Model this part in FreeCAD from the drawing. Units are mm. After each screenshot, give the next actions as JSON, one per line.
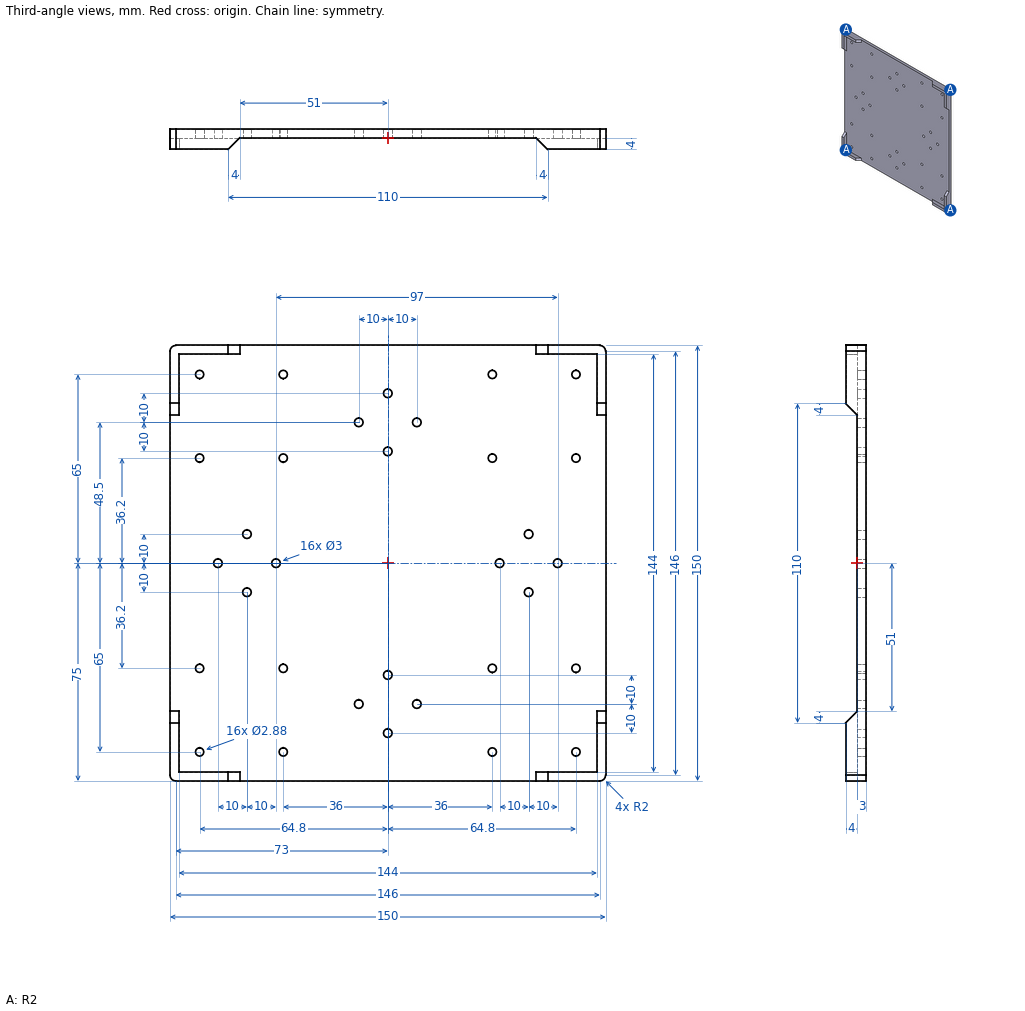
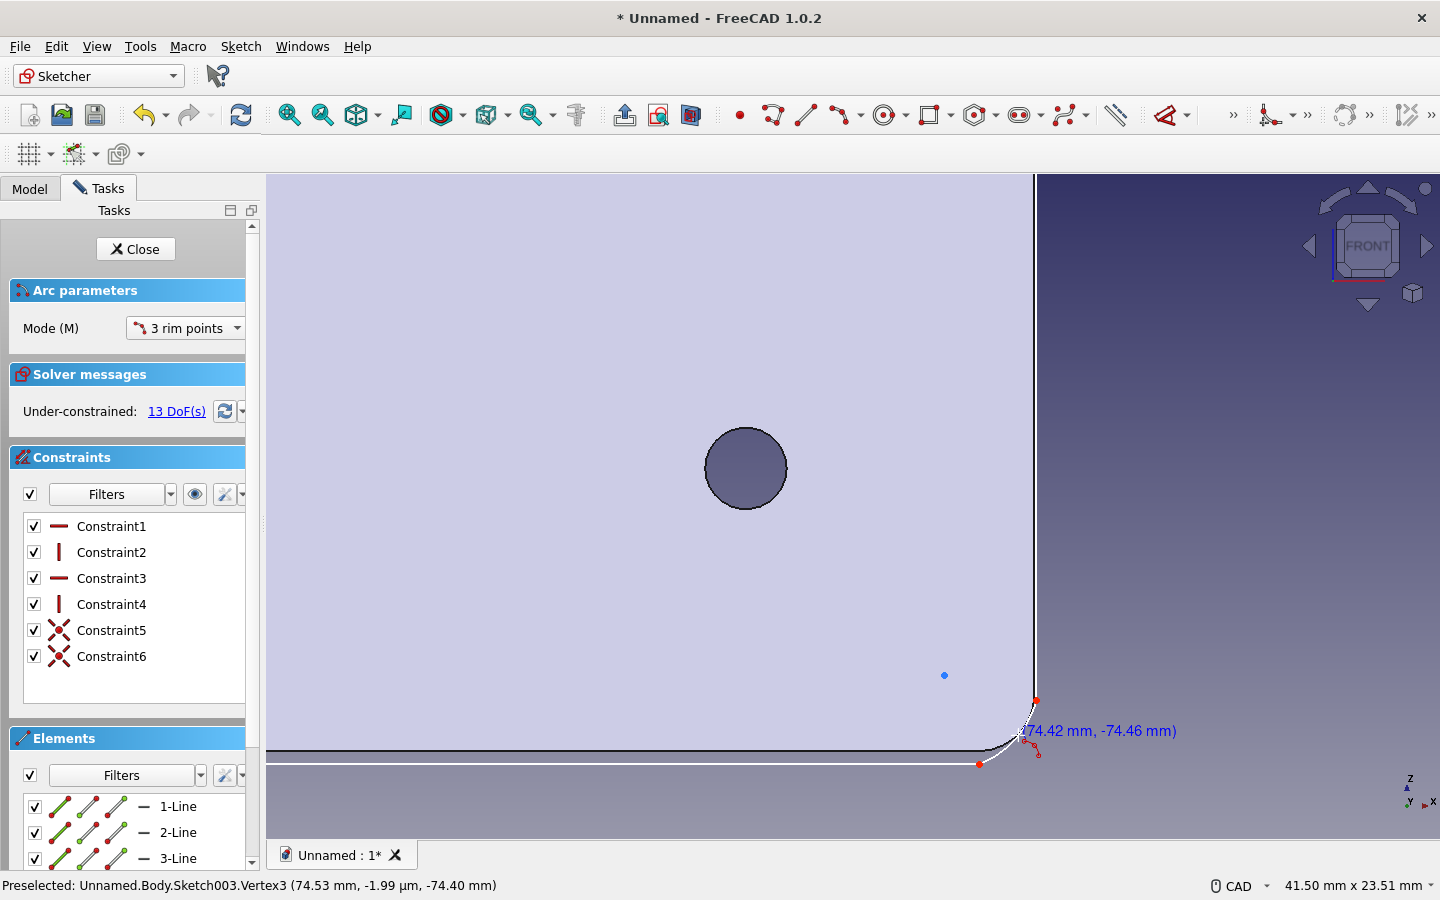
{"action": "scroll", "coordinate": [1018, 740], "scroll_direction": "down", "scroll_amount": 11}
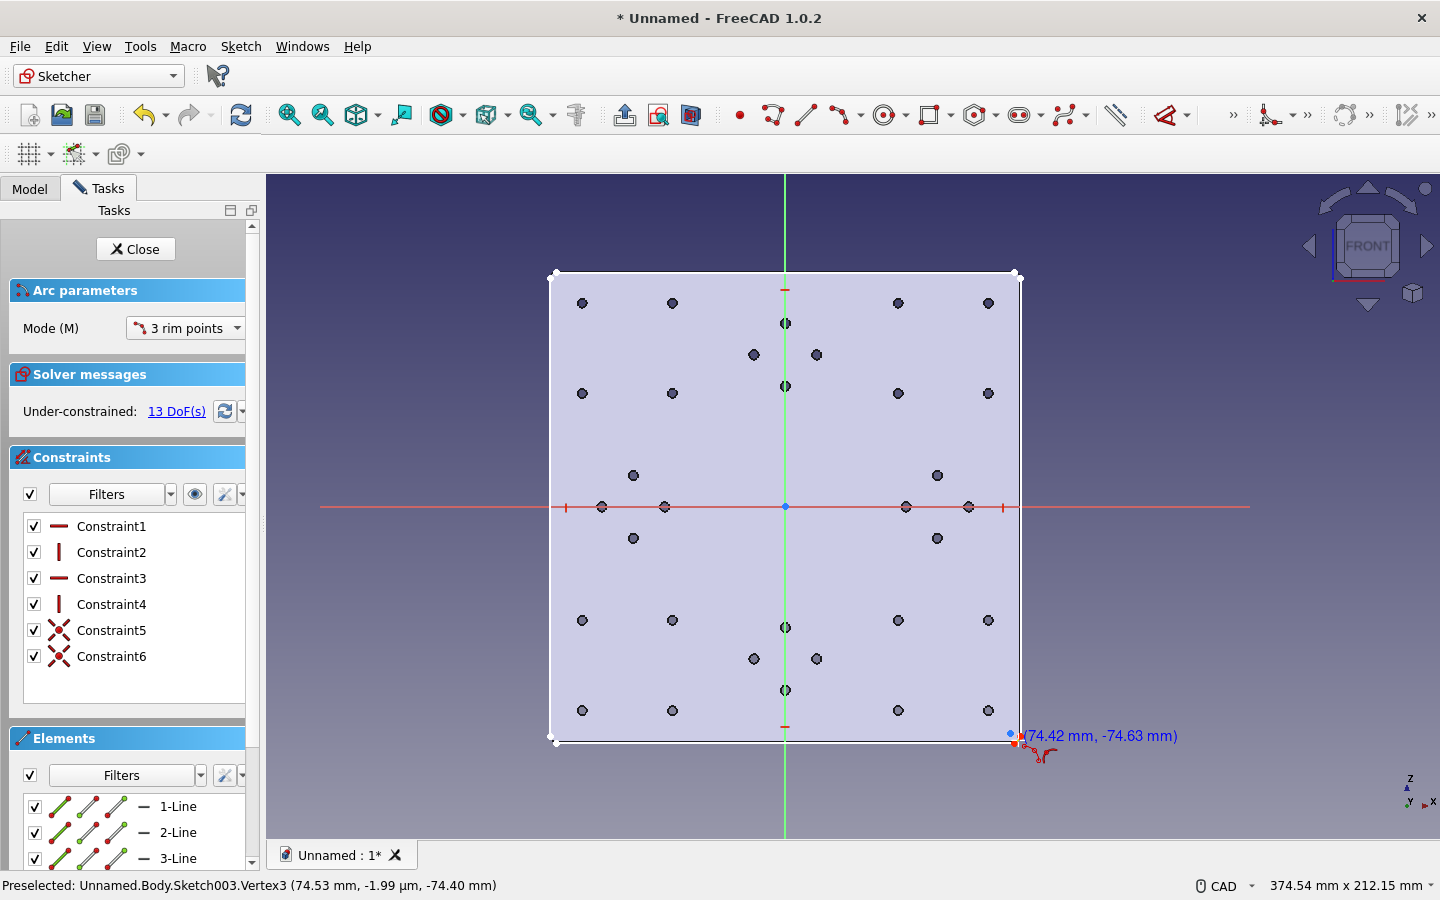
{"action": "scroll", "coordinate": [1020, 278], "scroll_direction": "up", "scroll_amount": 3}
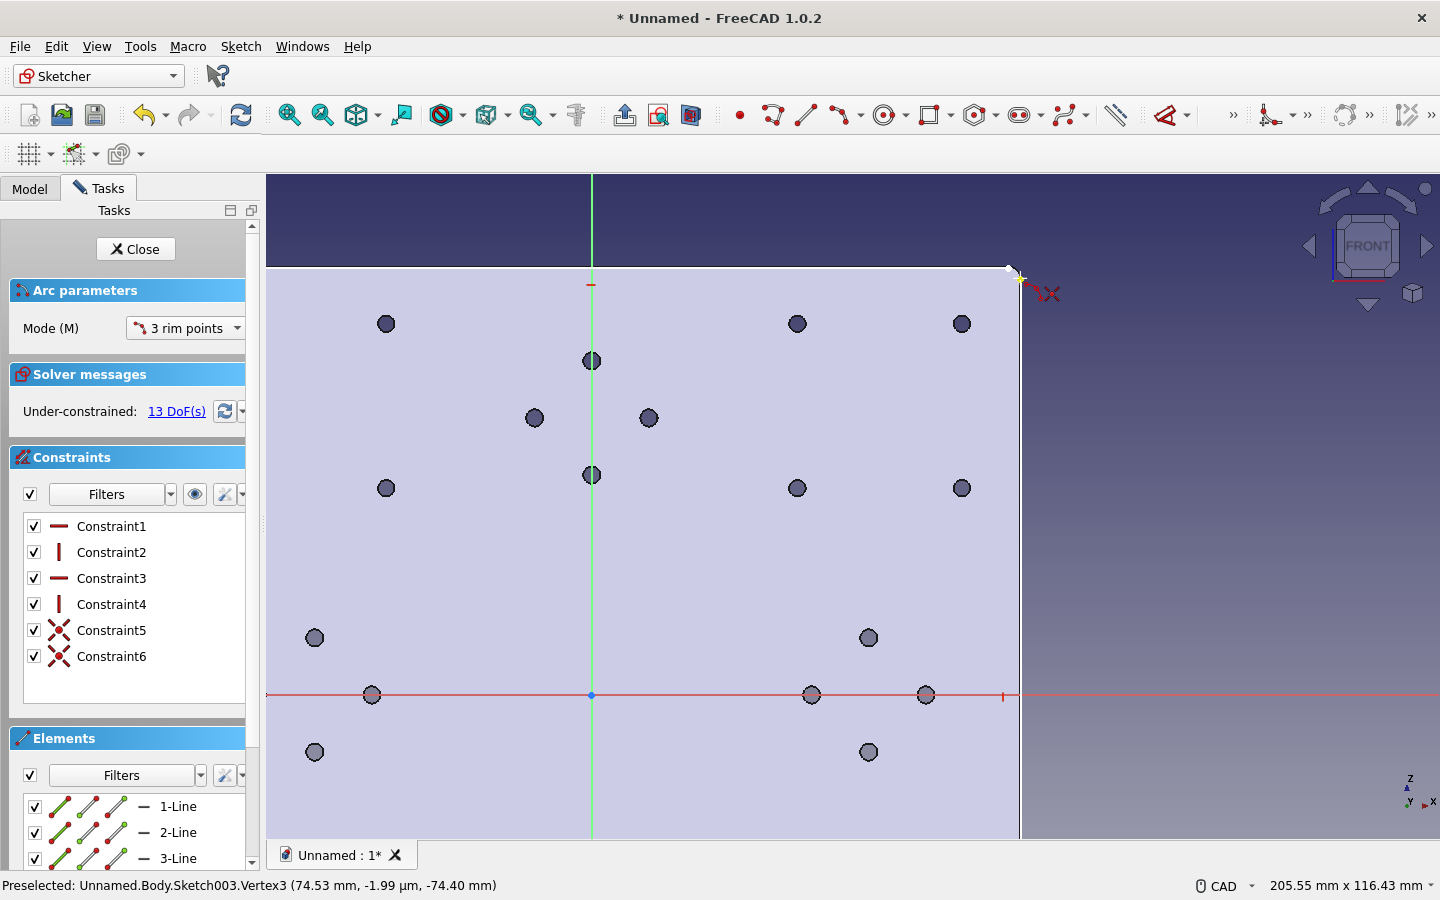
{"action": "left_click", "coordinate": [1021, 280]}
{"action": "left_click", "coordinate": [1009, 268]}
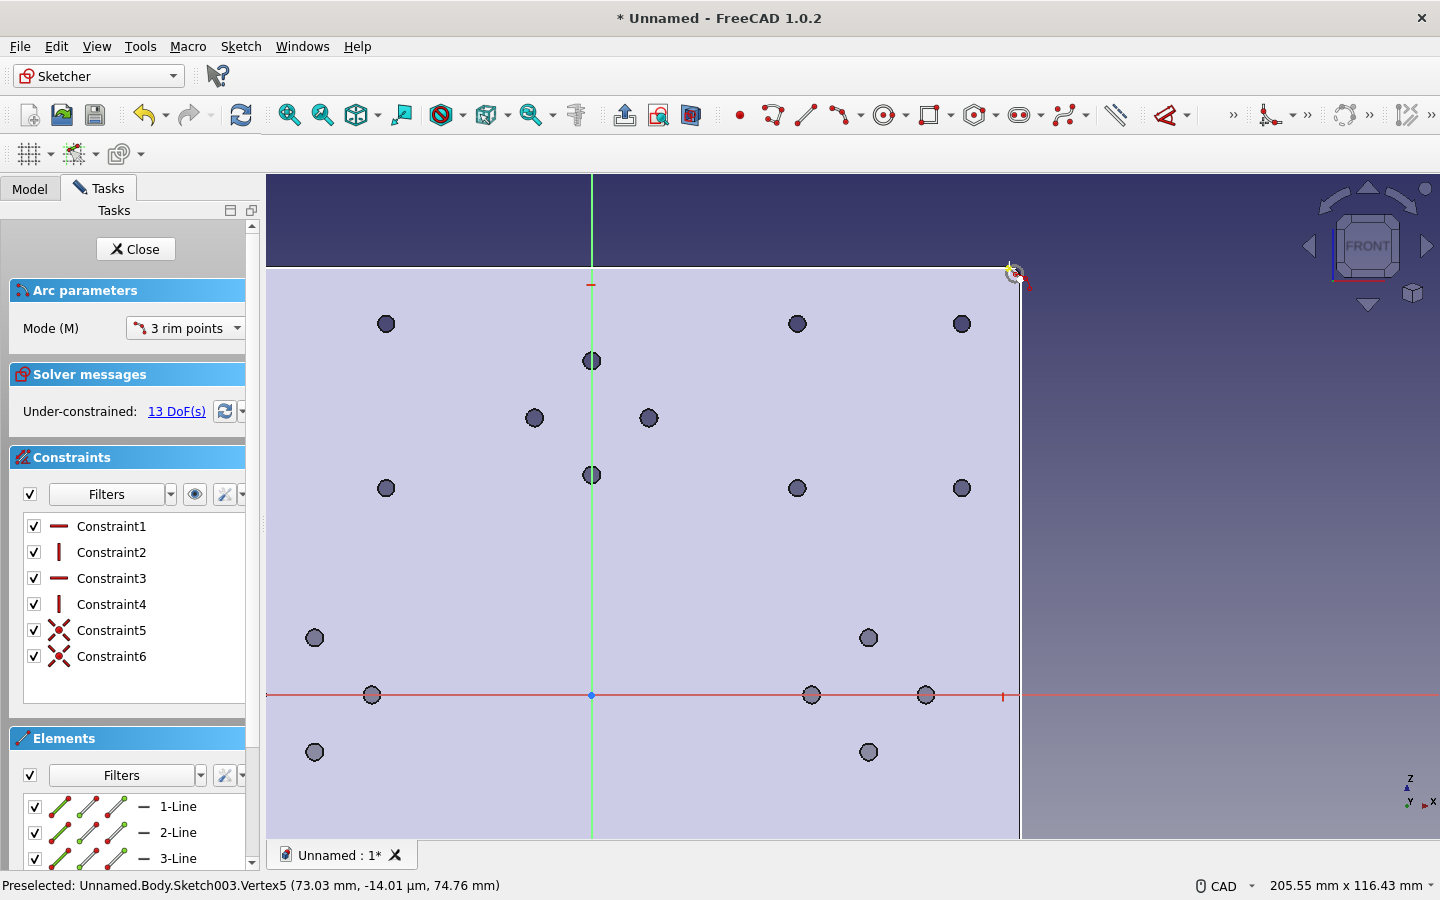
{"action": "scroll", "coordinate": [1017, 270], "scroll_direction": "up", "scroll_amount": 8}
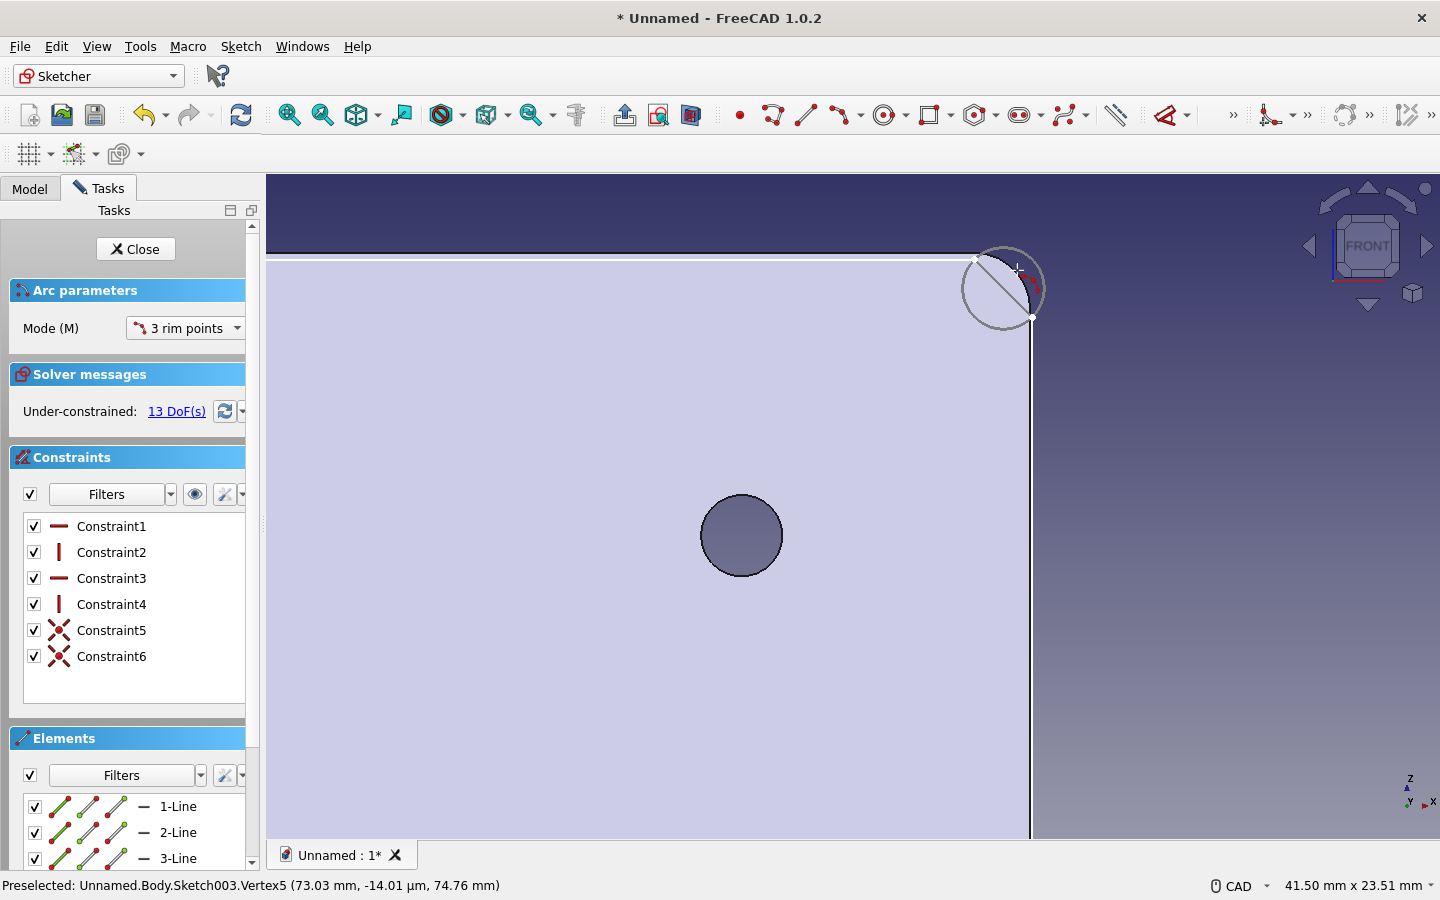
{"action": "left_click", "coordinate": [1014, 269]}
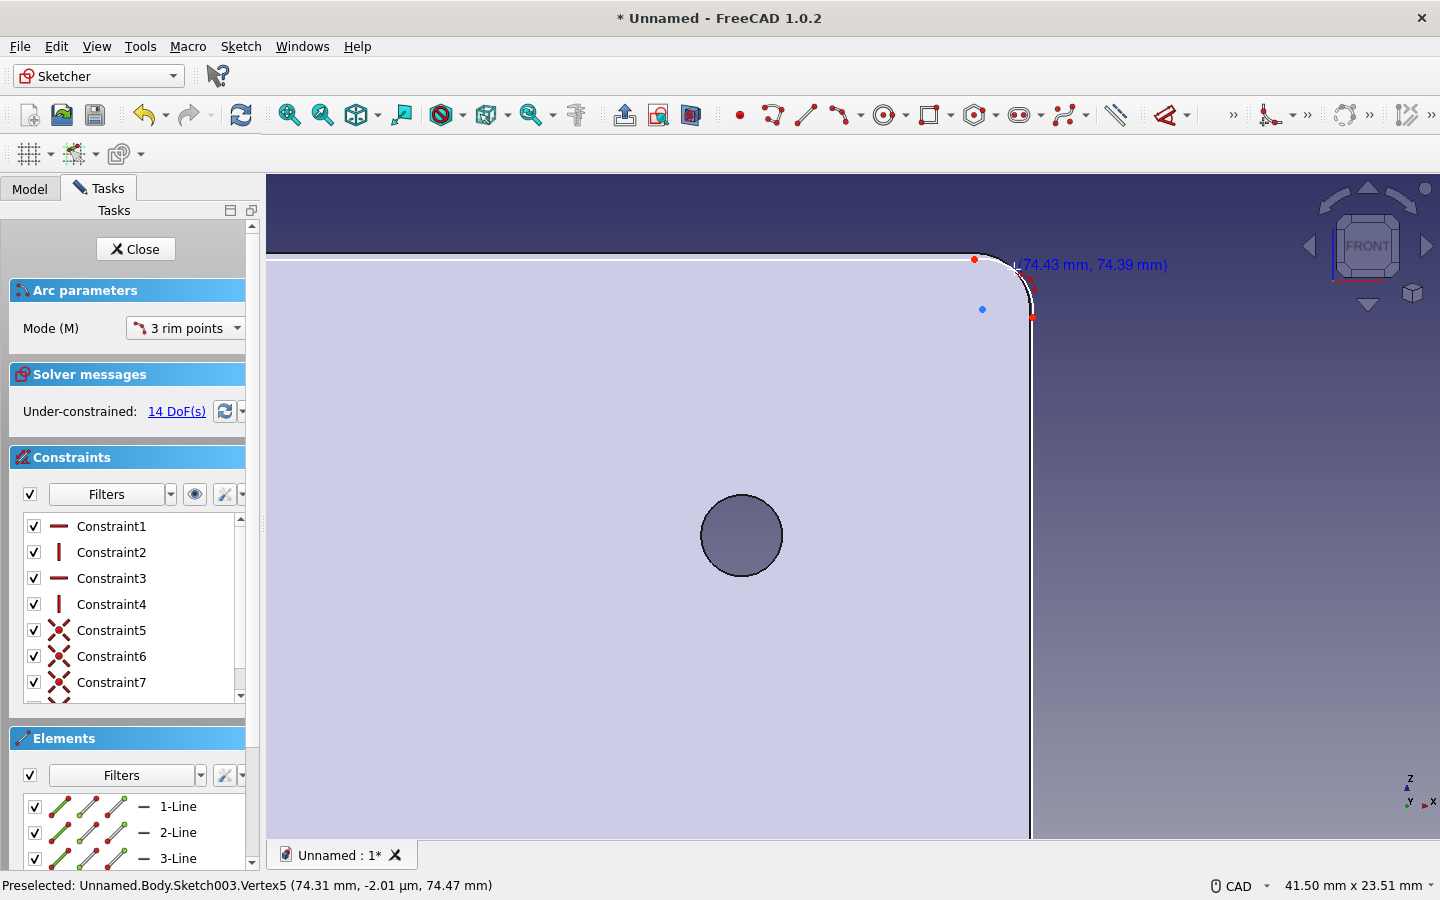
{"action": "scroll", "coordinate": [1018, 274], "scroll_direction": "down", "scroll_amount": 11}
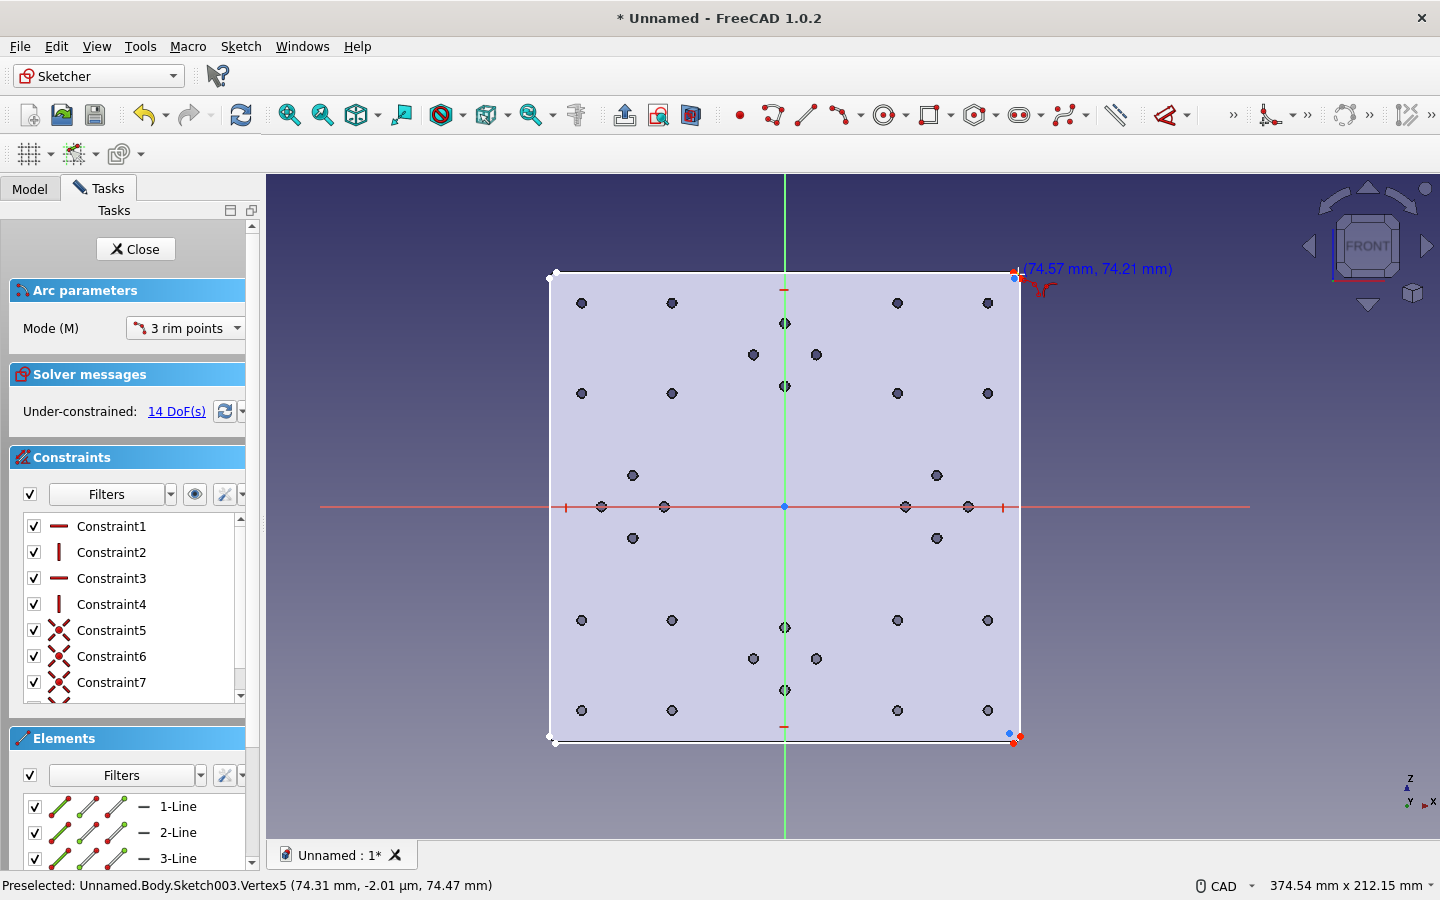
{"action": "scroll", "coordinate": [556, 272], "scroll_direction": "up", "scroll_amount": 3}